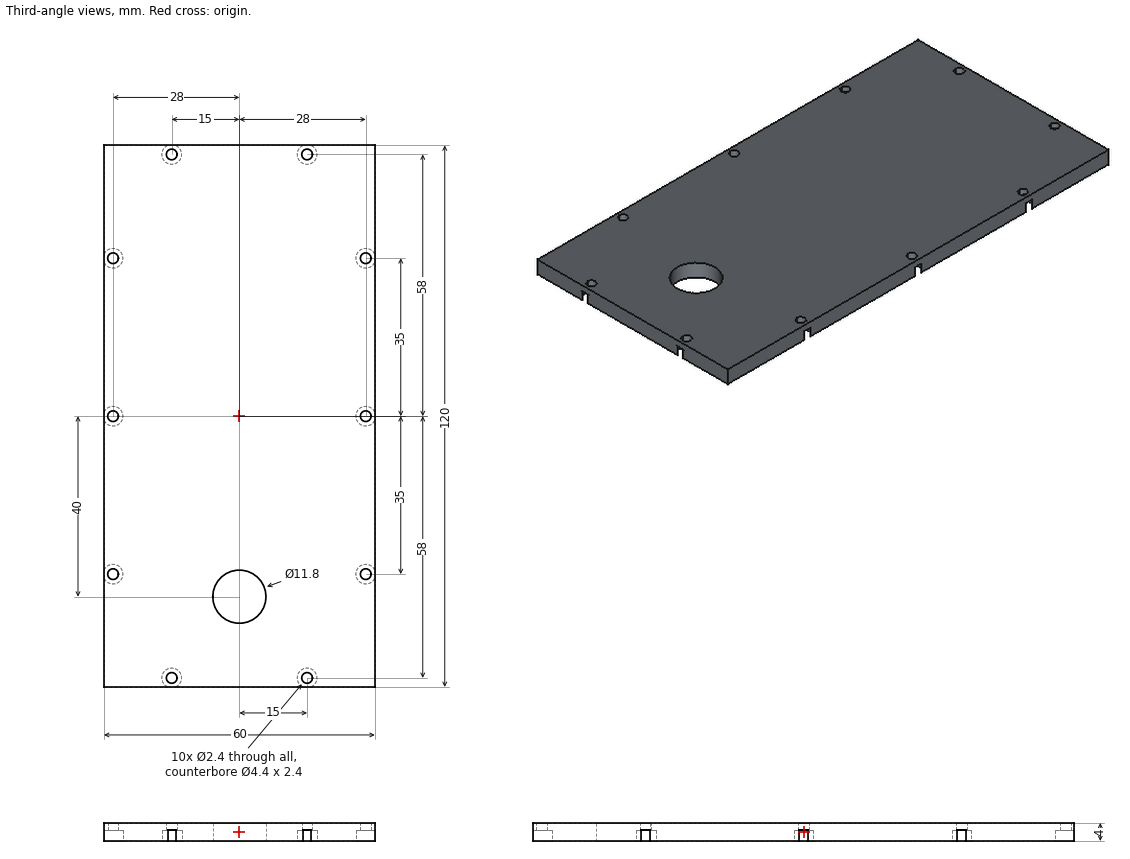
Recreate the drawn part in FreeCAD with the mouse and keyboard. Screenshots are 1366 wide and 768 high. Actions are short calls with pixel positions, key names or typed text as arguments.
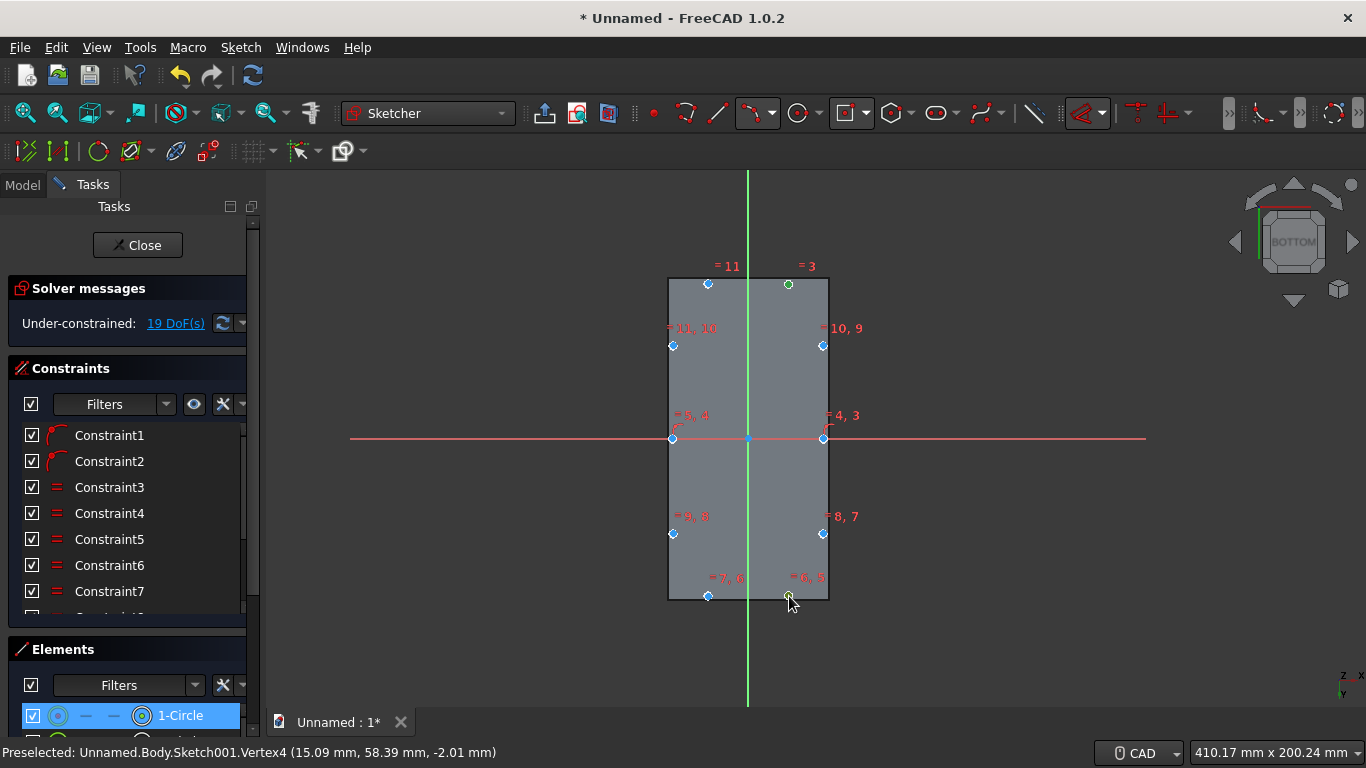
click(1190, 114)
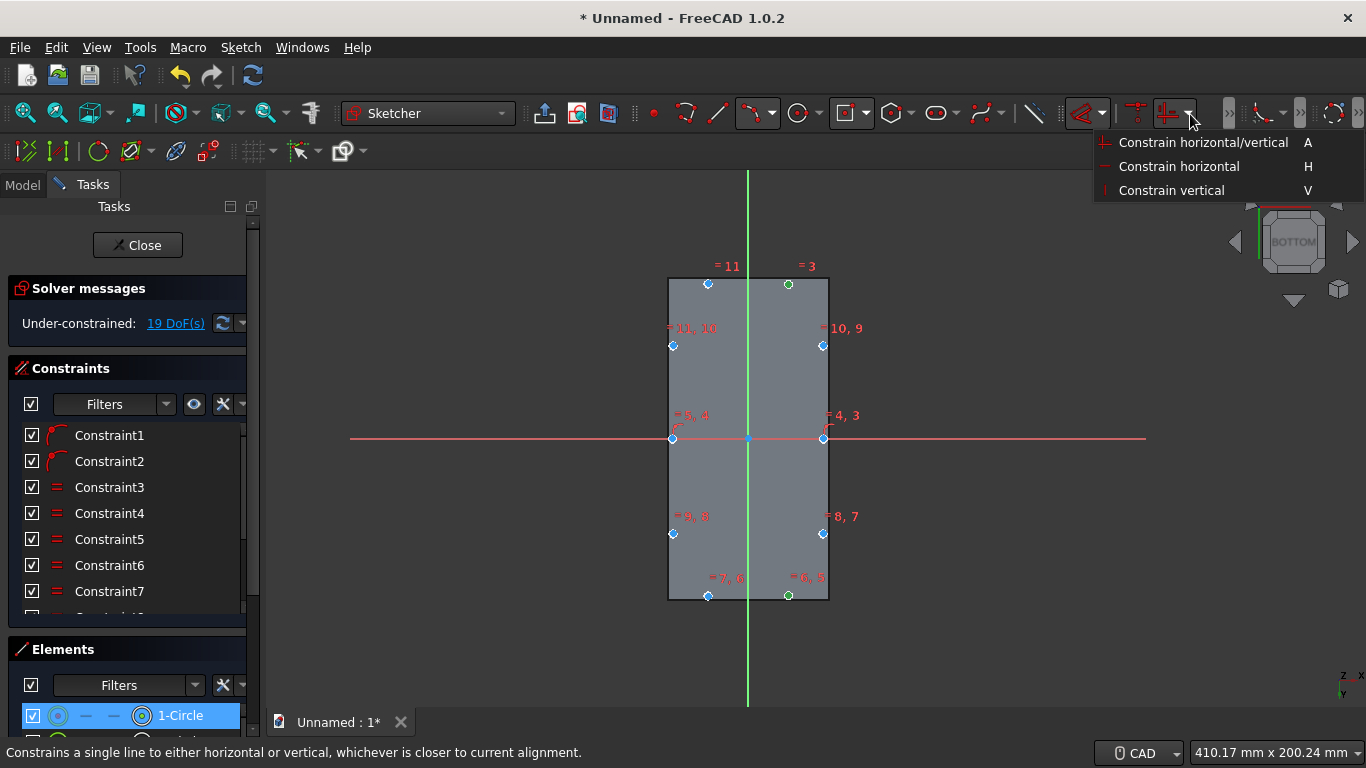
click(1229, 190)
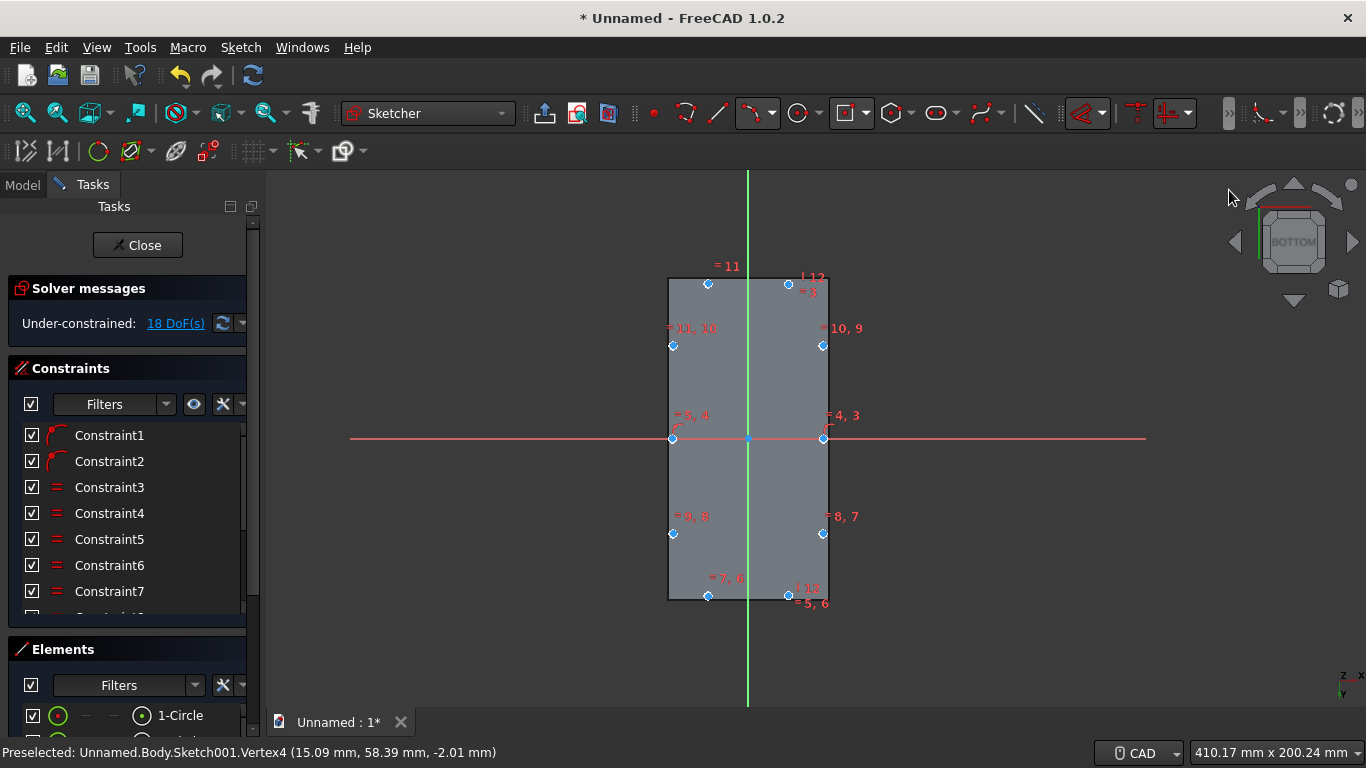
click(789, 596)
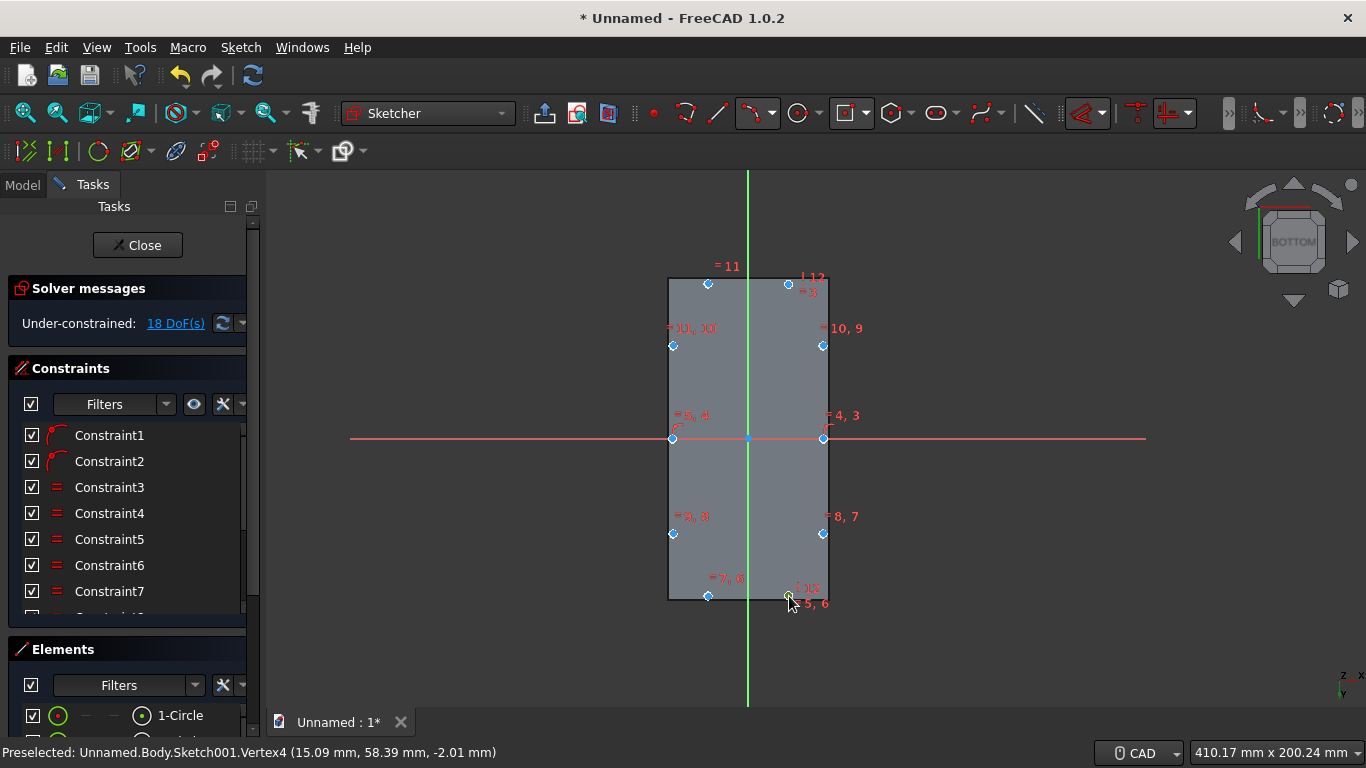
click(708, 596)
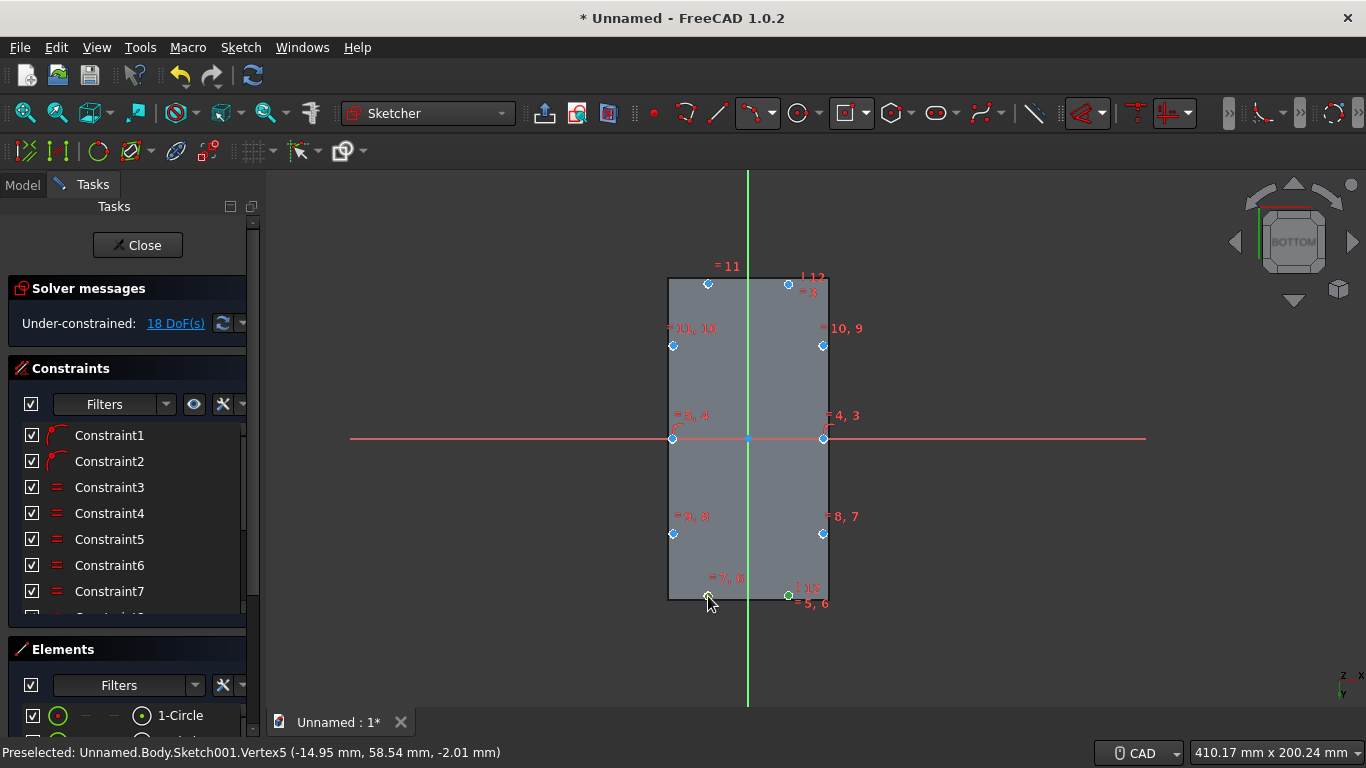
click(1190, 114)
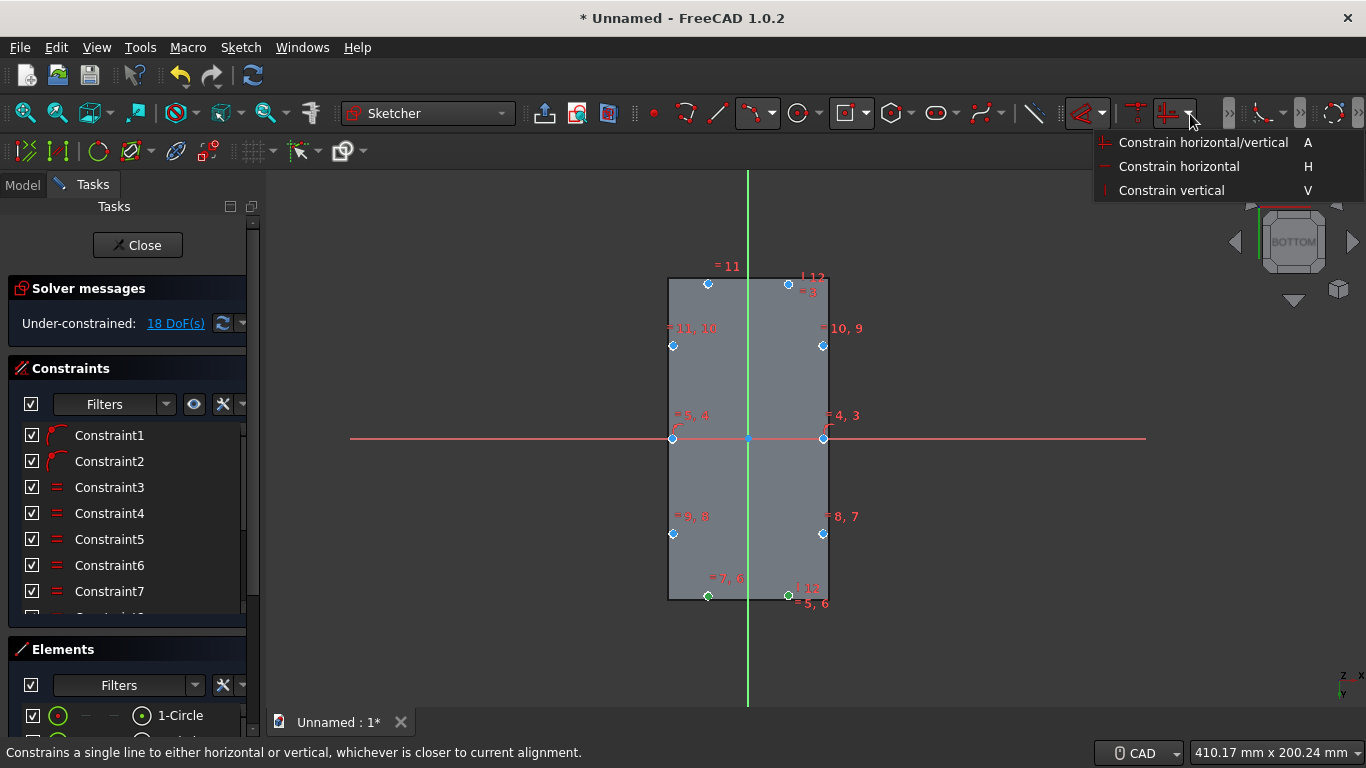
click(1229, 166)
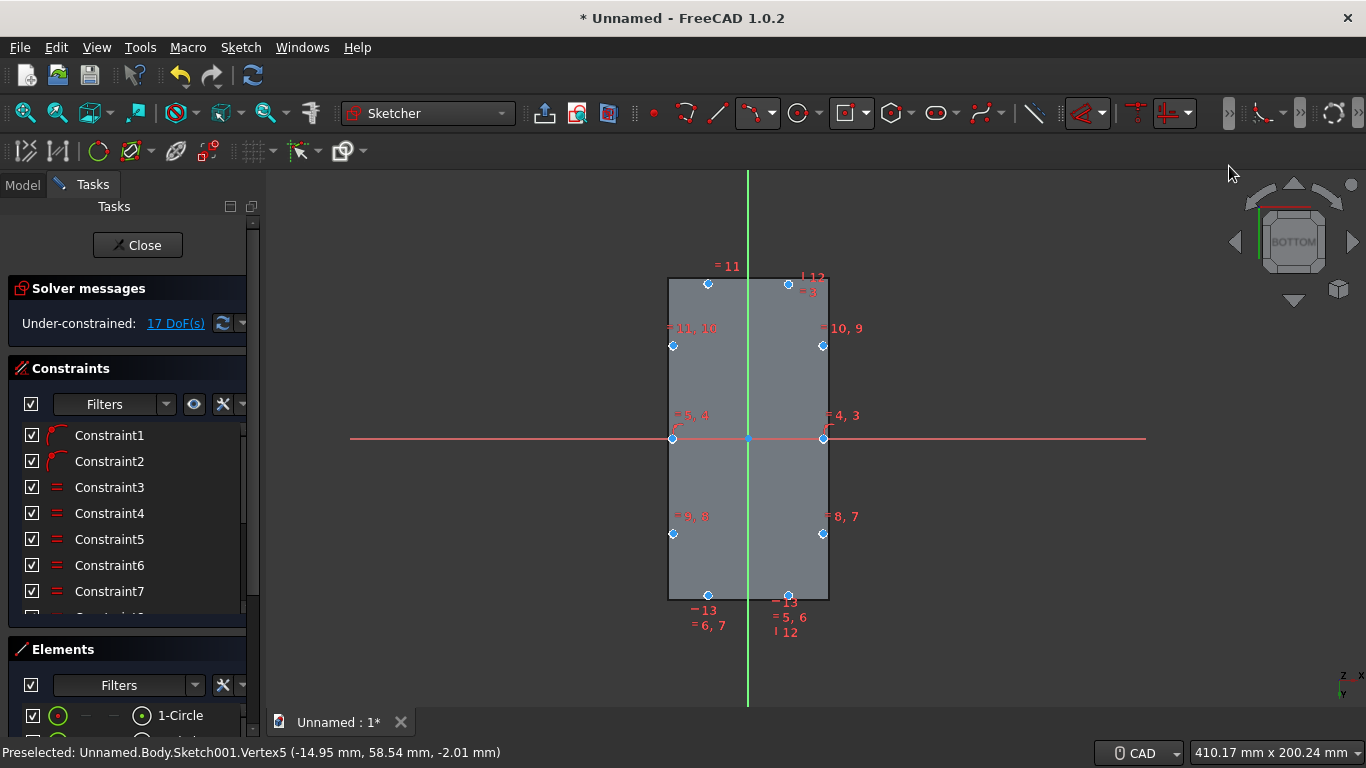
click(824, 439)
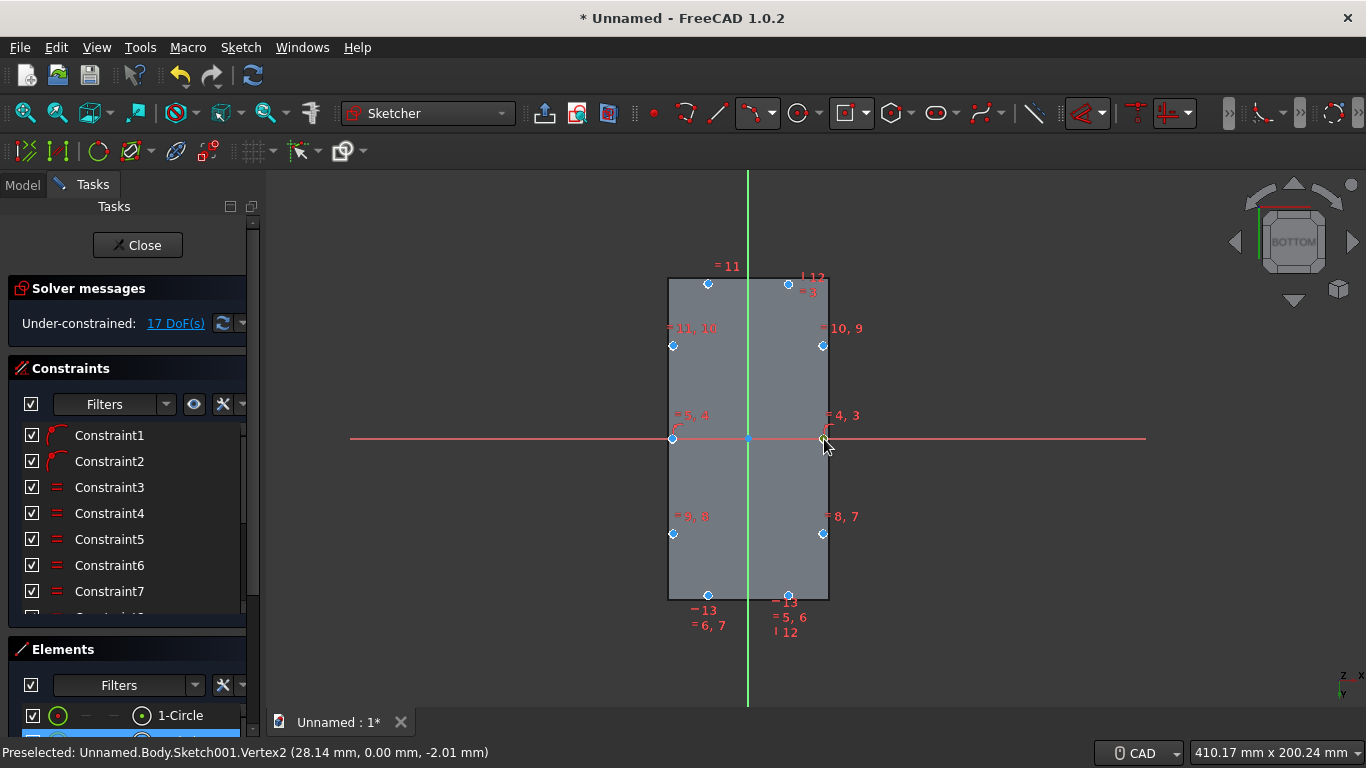
click(823, 534)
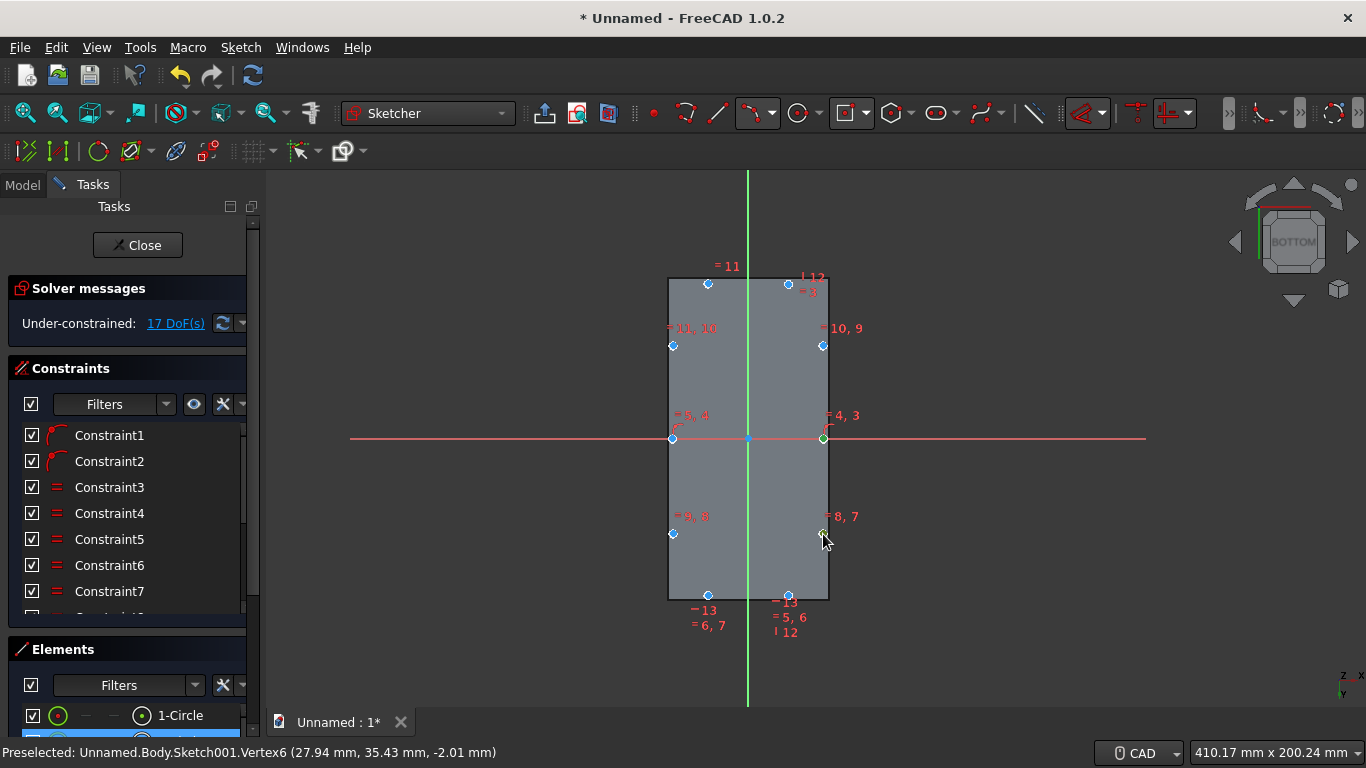
key(v)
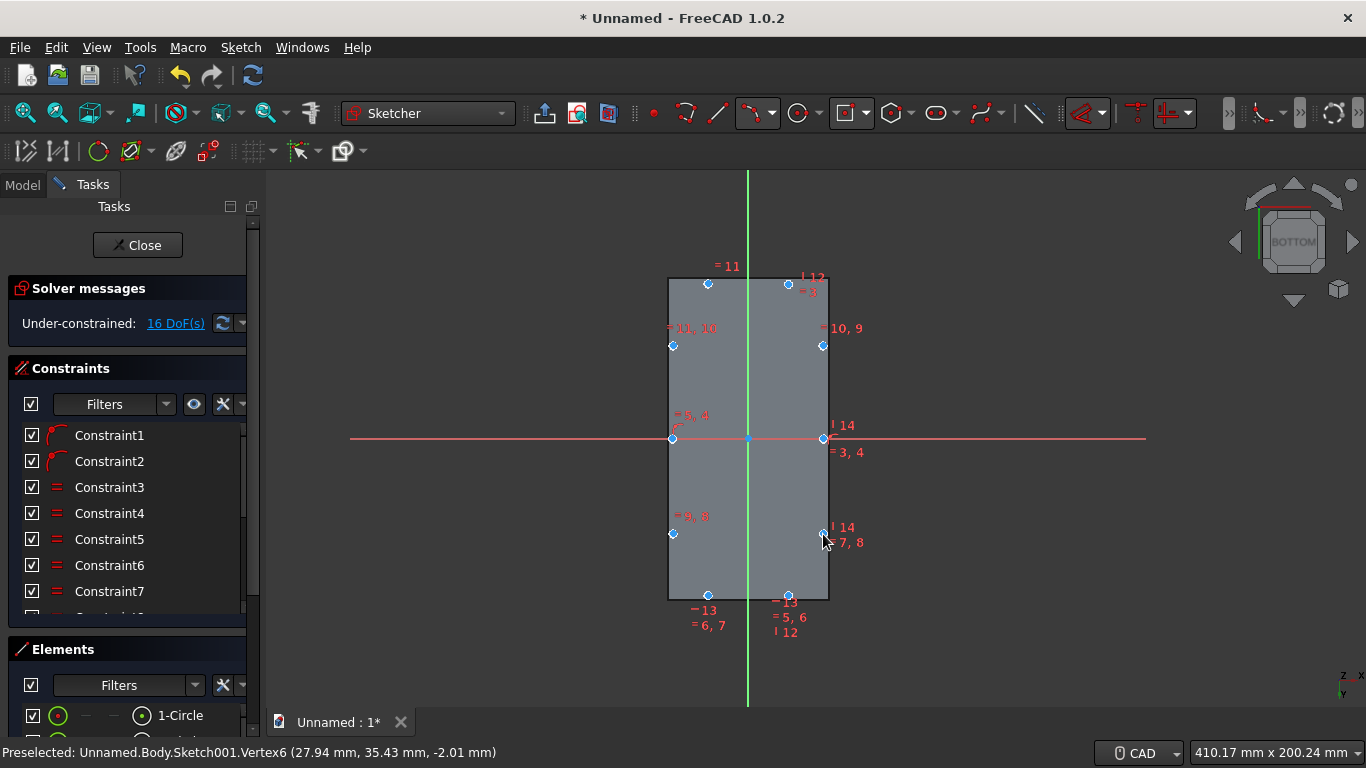
click(673, 439)